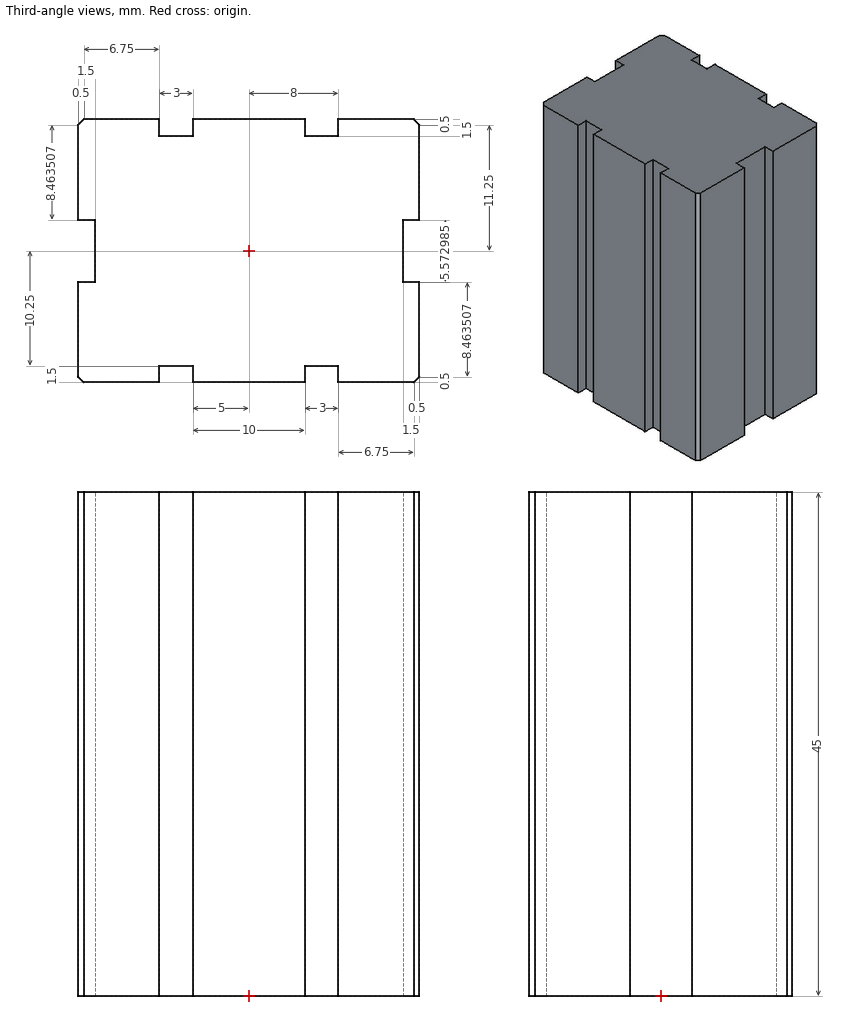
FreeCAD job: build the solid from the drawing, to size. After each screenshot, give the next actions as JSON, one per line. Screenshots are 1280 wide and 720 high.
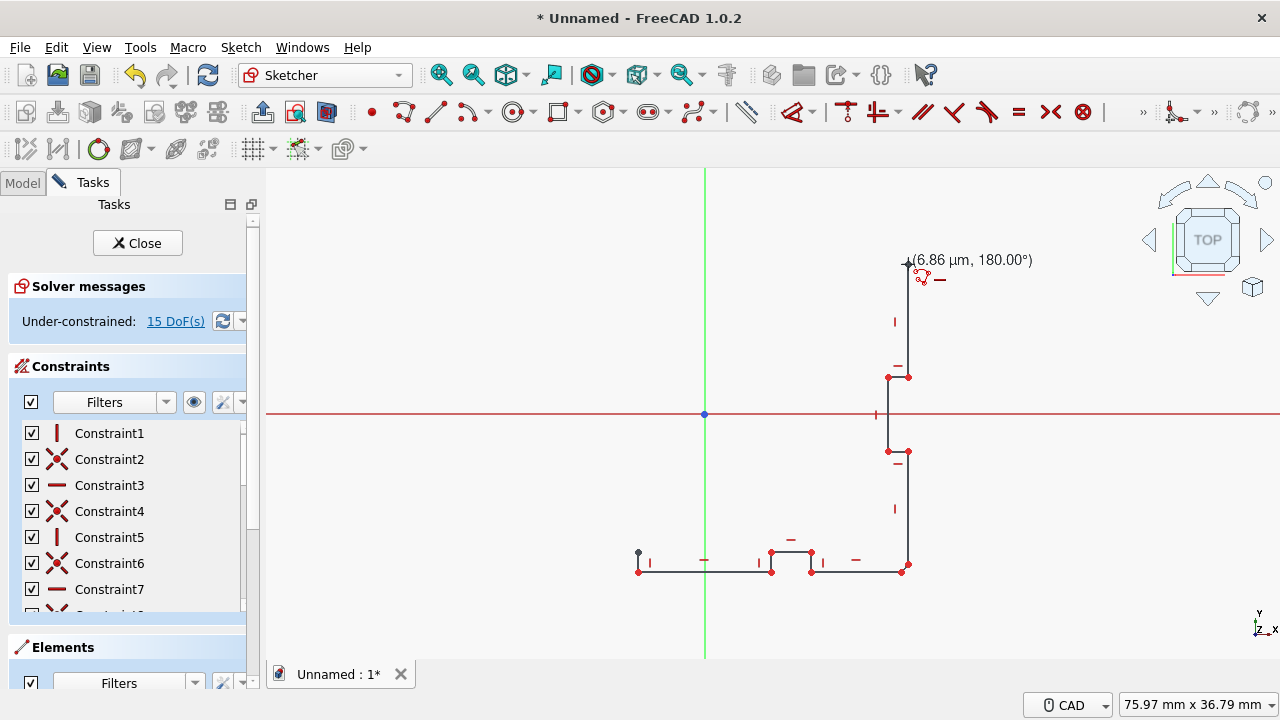
{"action": "scroll", "coordinate": [902, 257], "scroll_direction": "up", "scroll_amount": 3}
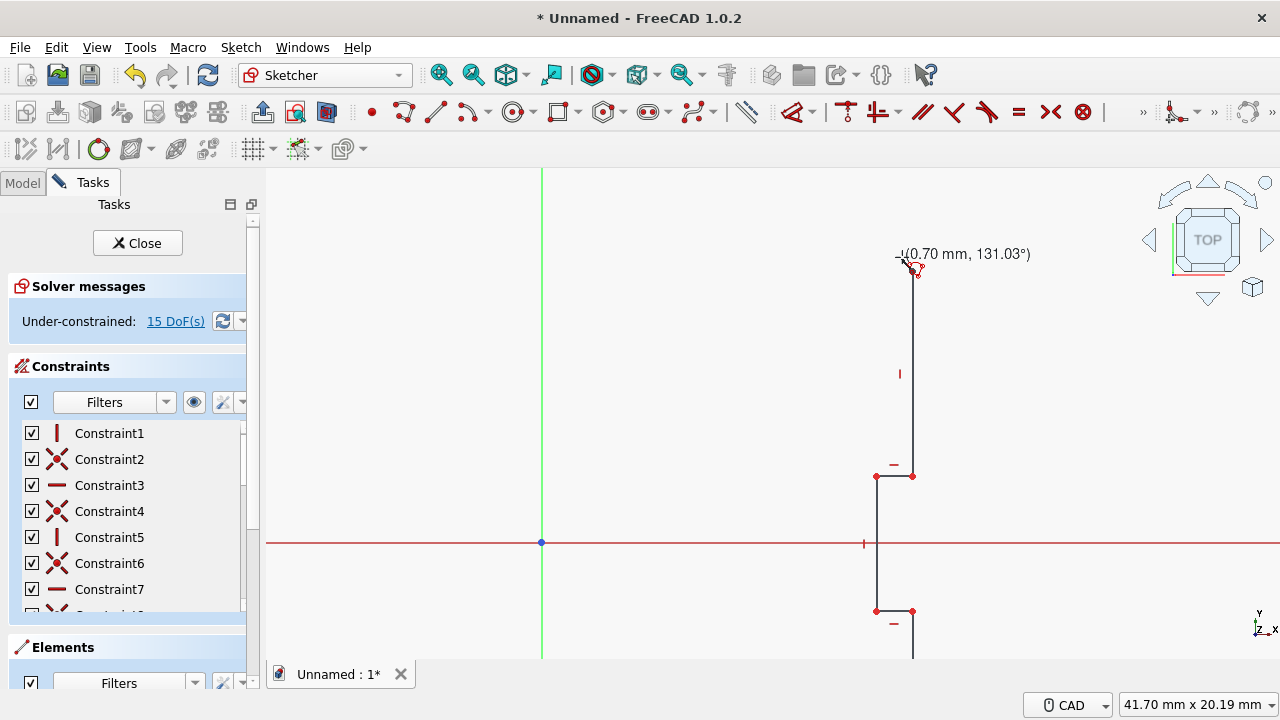
{"action": "left_click", "coordinate": [901, 257]}
{"action": "left_click", "coordinate": [737, 257]}
{"action": "left_click", "coordinate": [737, 294]}
{"action": "left_click", "coordinate": [664, 294]}
{"action": "left_click", "coordinate": [664, 257]}
{"action": "left_click", "coordinate": [420, 257]}
{"action": "left_click", "coordinate": [420, 294]}
{"action": "left_click", "coordinate": [347, 294]}
{"action": "left_click", "coordinate": [347, 257]}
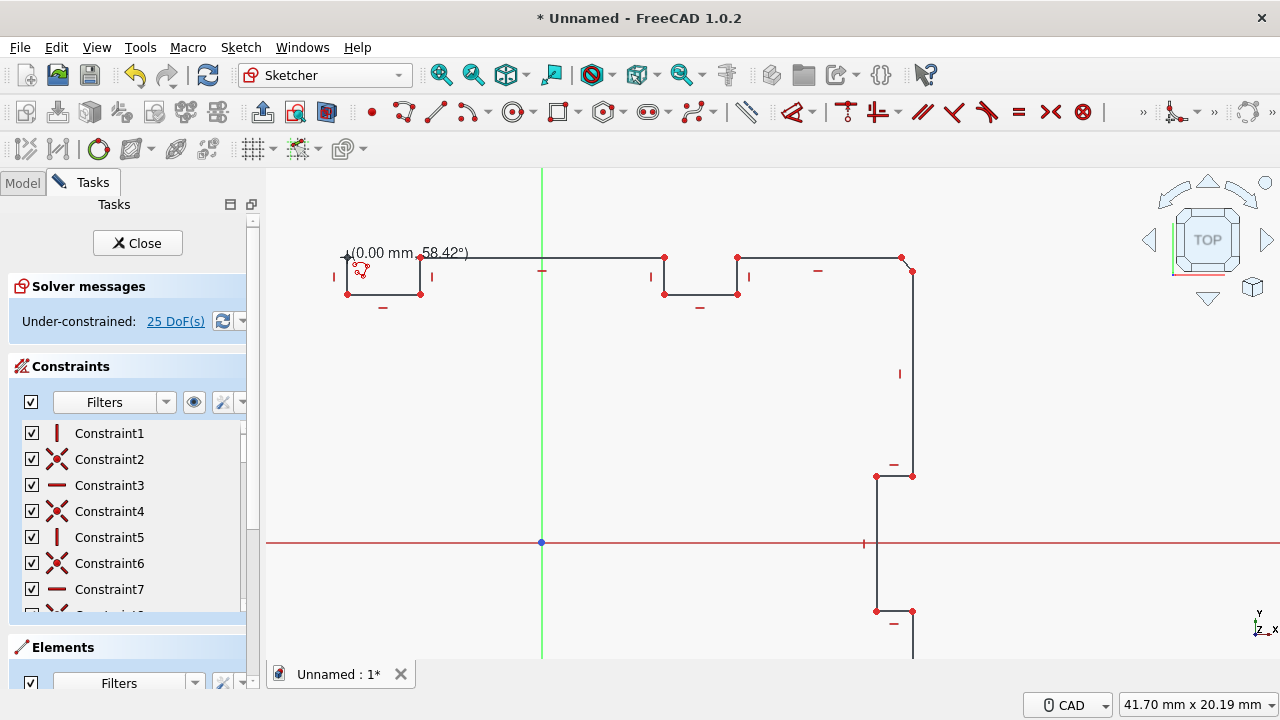
{"action": "scroll", "coordinate": [902, 256], "scroll_direction": "down", "scroll_amount": 3}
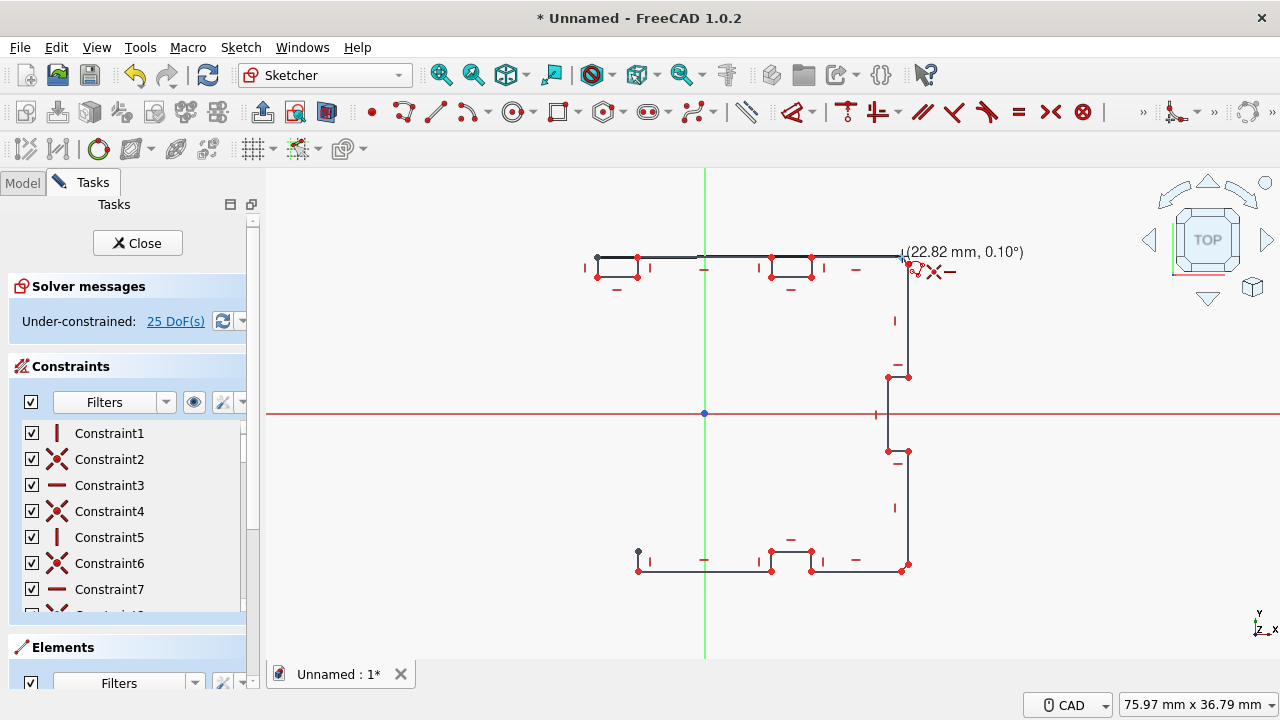
{"action": "left_click", "coordinate": [508, 257]}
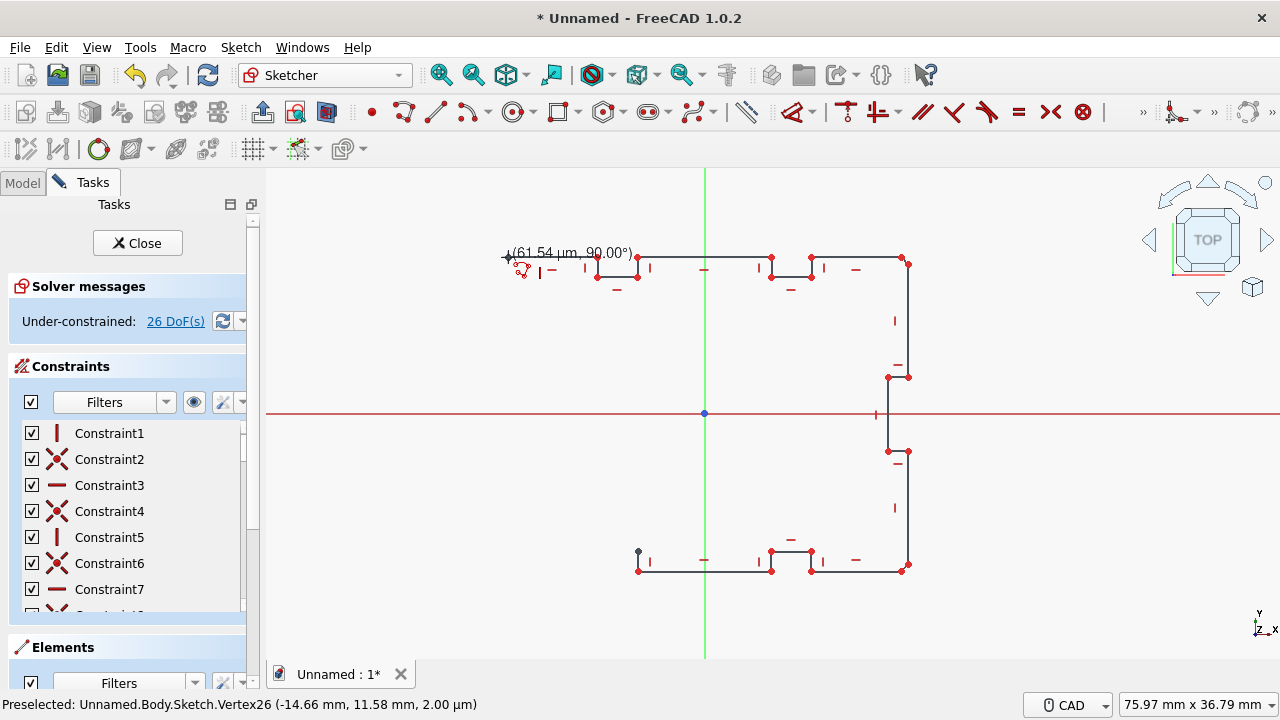
{"action": "scroll", "coordinate": [501, 263], "scroll_direction": "up", "scroll_amount": 3}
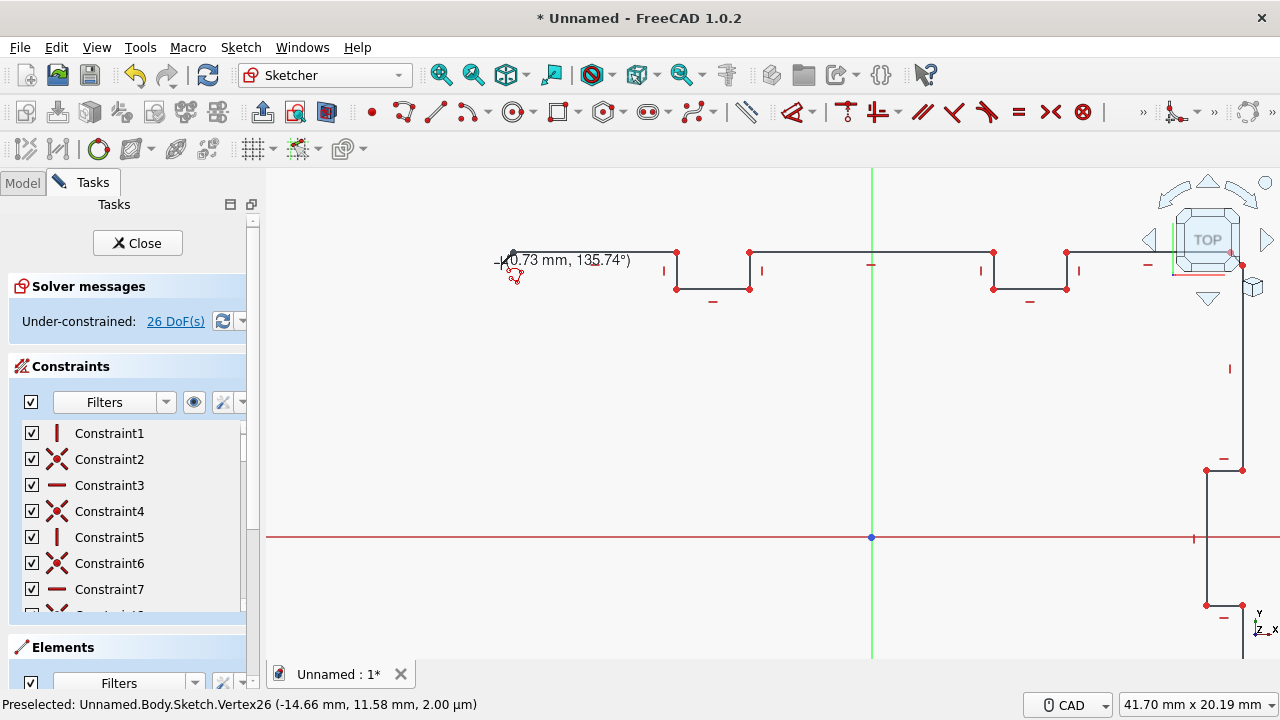
{"action": "left_click", "coordinate": [501, 264]}
{"action": "left_click", "coordinate": [501, 469]}
{"action": "left_click", "coordinate": [538, 469]}
{"action": "left_click", "coordinate": [538, 605]}
{"action": "left_click", "coordinate": [501, 605]}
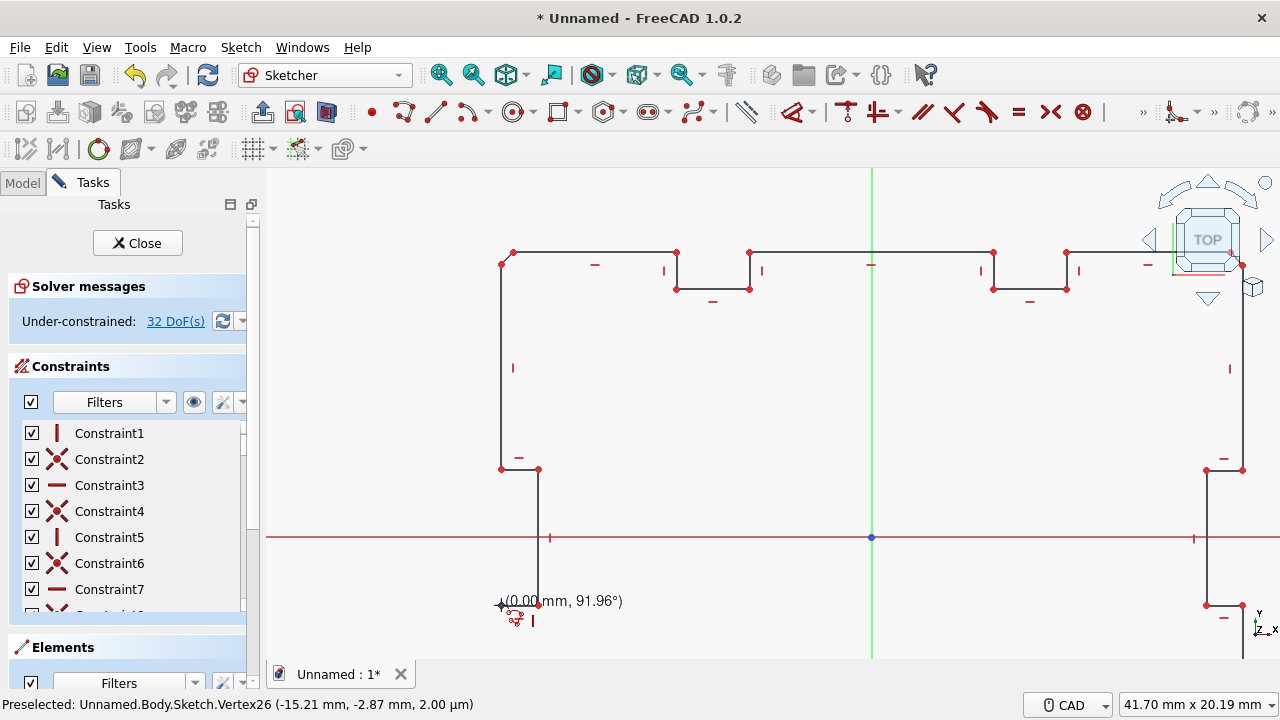
{"action": "scroll", "coordinate": [501, 263], "scroll_direction": "down", "scroll_amount": 3}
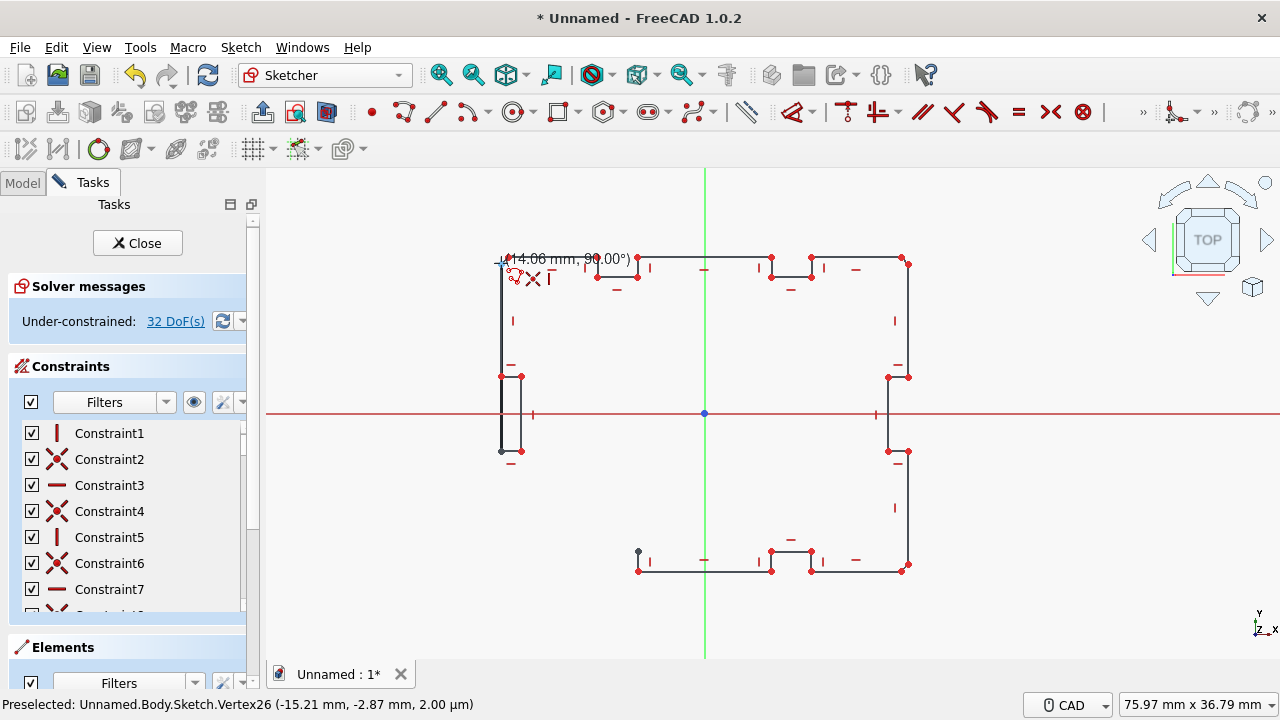
{"action": "left_click", "coordinate": [501, 564]}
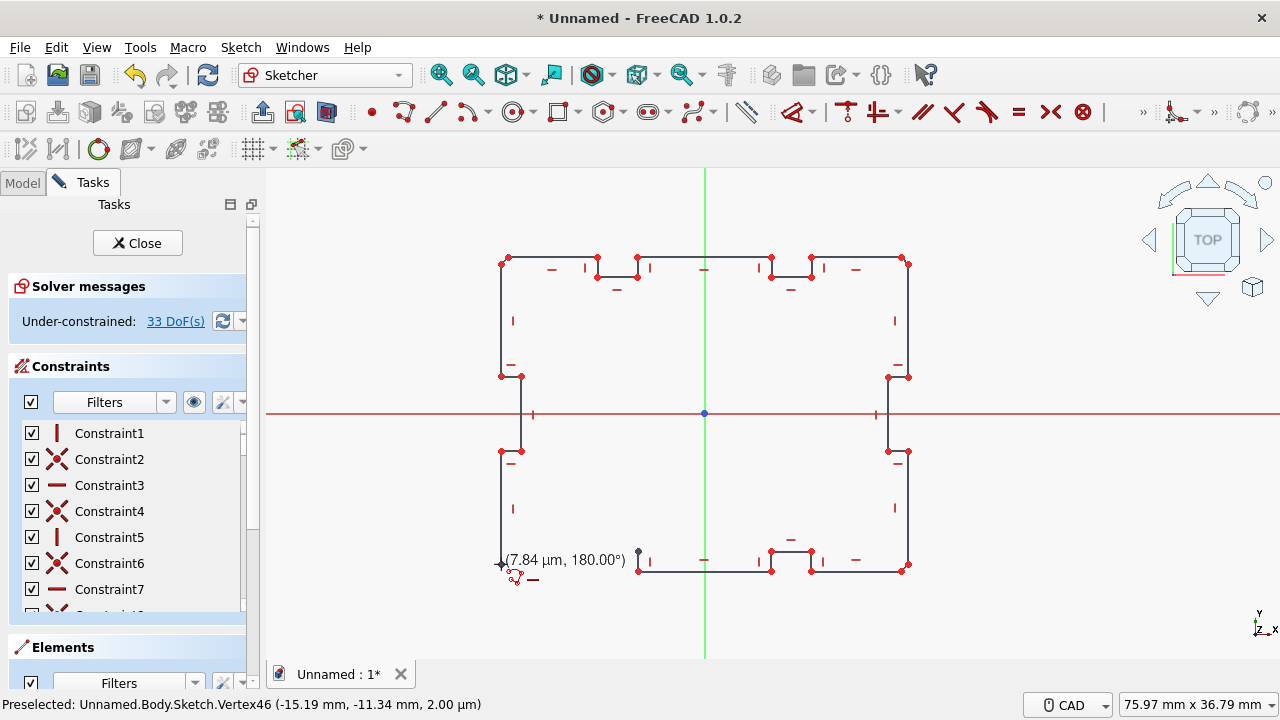
{"action": "scroll", "coordinate": [508, 570], "scroll_direction": "up", "scroll_amount": 3}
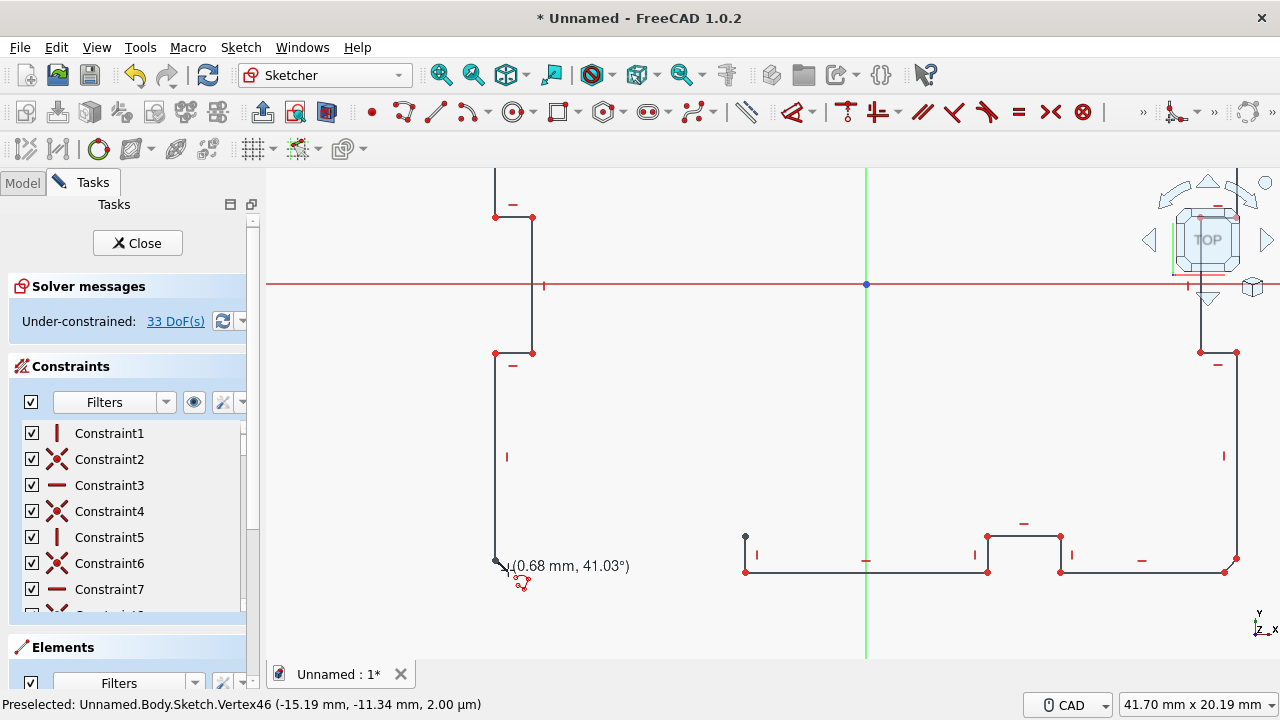
{"action": "left_click", "coordinate": [507, 570]}
{"action": "left_click", "coordinate": [672, 570]}
{"action": "left_click", "coordinate": [672, 534]}
{"action": "left_click", "coordinate": [745, 536]}
{"action": "key", "text": "Escape"}
{"action": "key", "text": "Escape"}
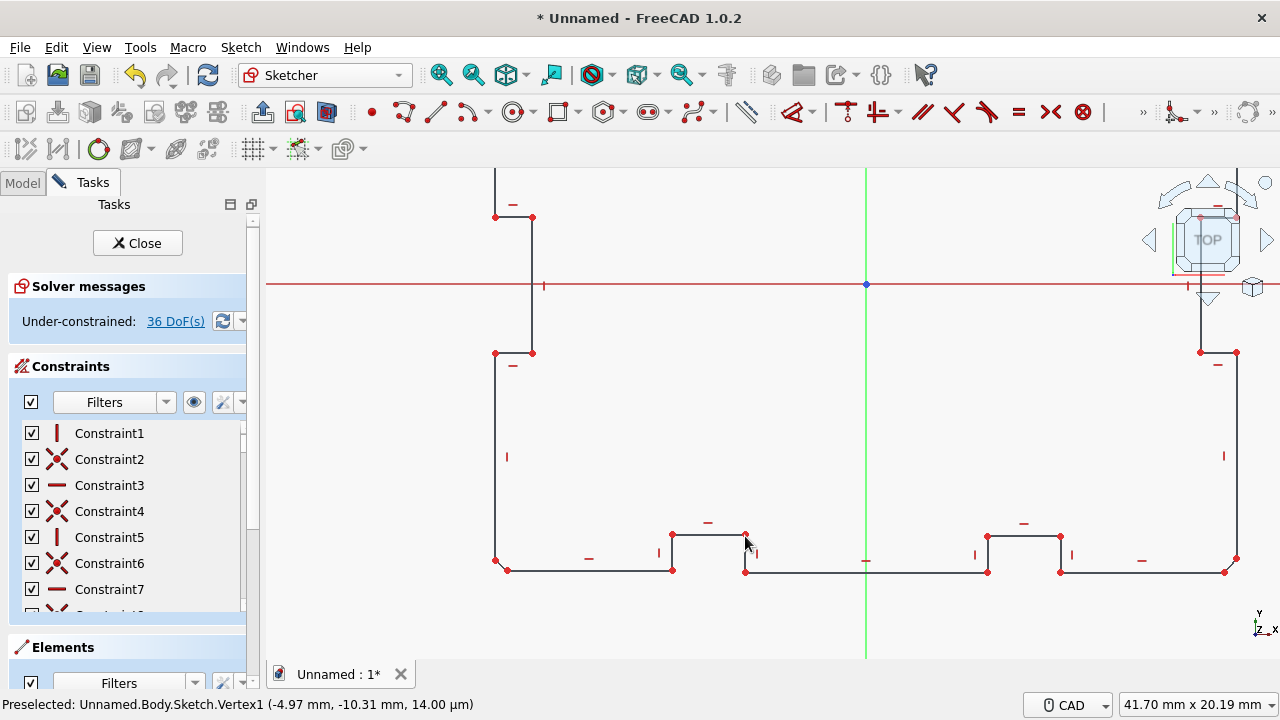
{"action": "key", "text": "d"}